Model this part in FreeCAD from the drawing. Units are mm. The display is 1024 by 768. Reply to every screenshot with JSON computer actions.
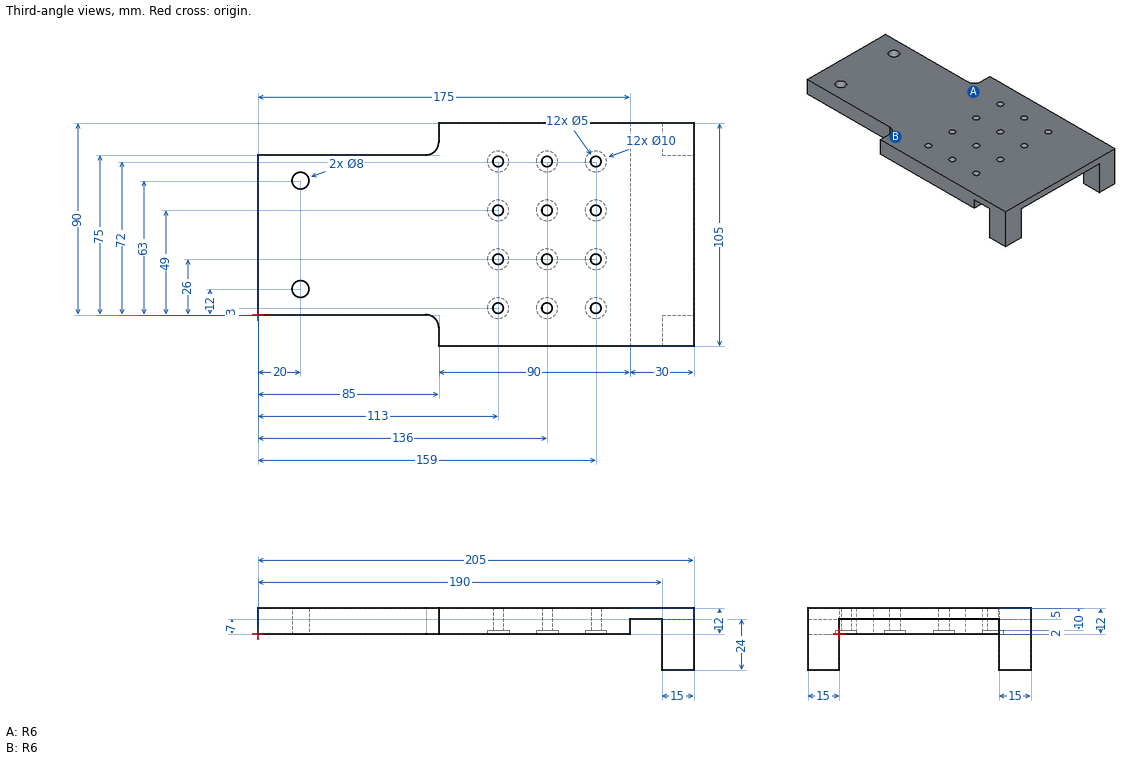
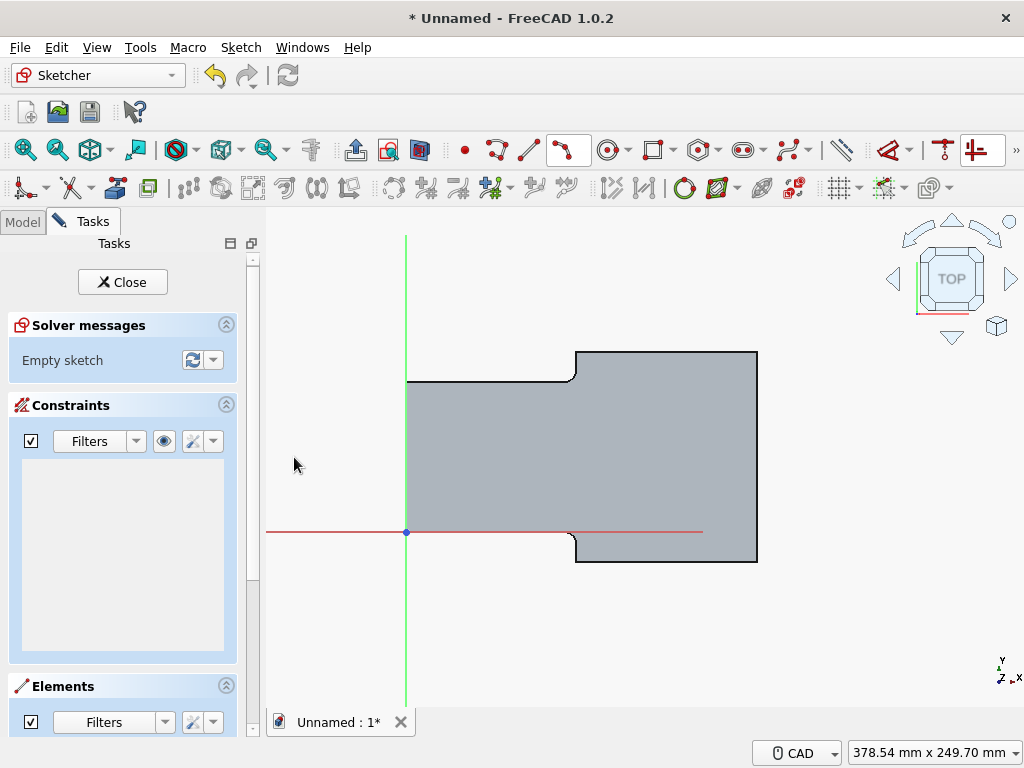
{"action": "left_click", "coordinate": [654, 150]}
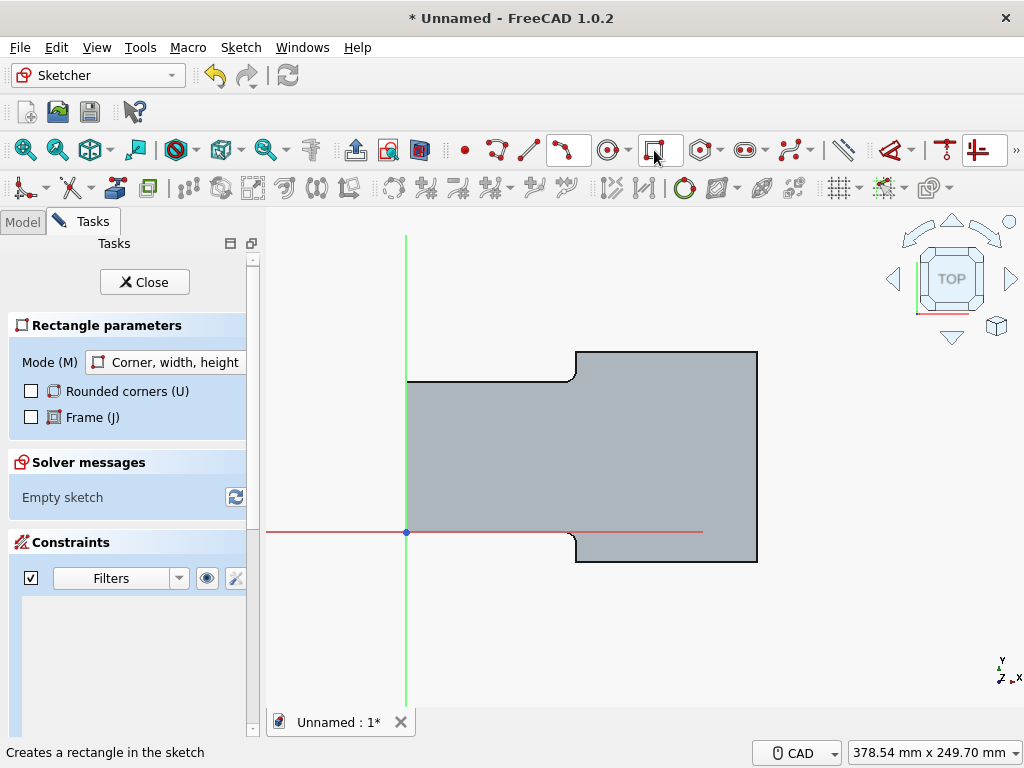
{"action": "left_click", "coordinate": [757, 352]}
{"action": "mouse_move", "coordinate": [817, 562]}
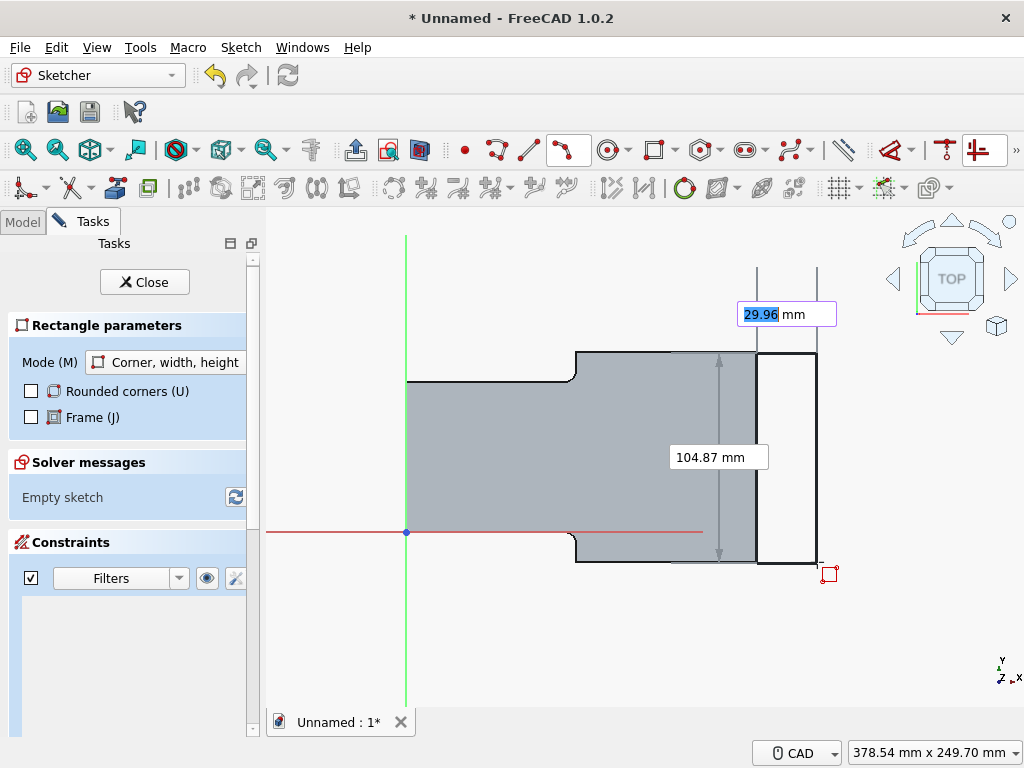
{"action": "type", "text": "30"}
{"action": "key", "text": "Tab"}
{"action": "type", "text": "105"}
{"action": "key", "text": "Return"}
{"action": "key", "text": "Escape"}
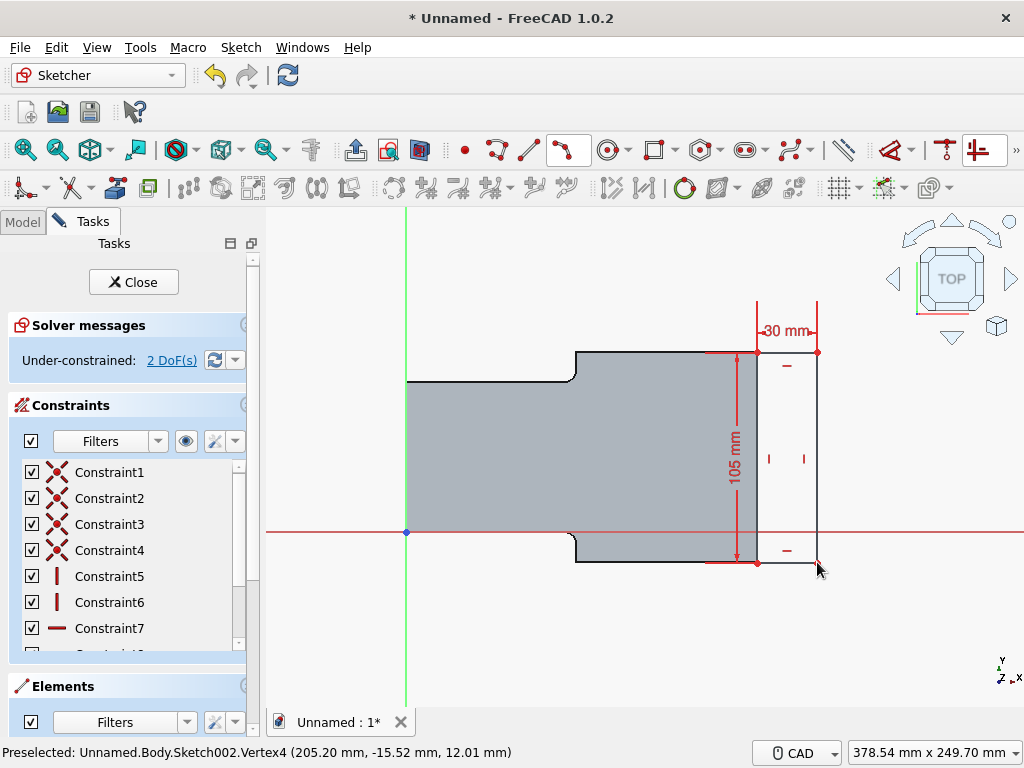
{"action": "left_click", "coordinate": [890, 150]}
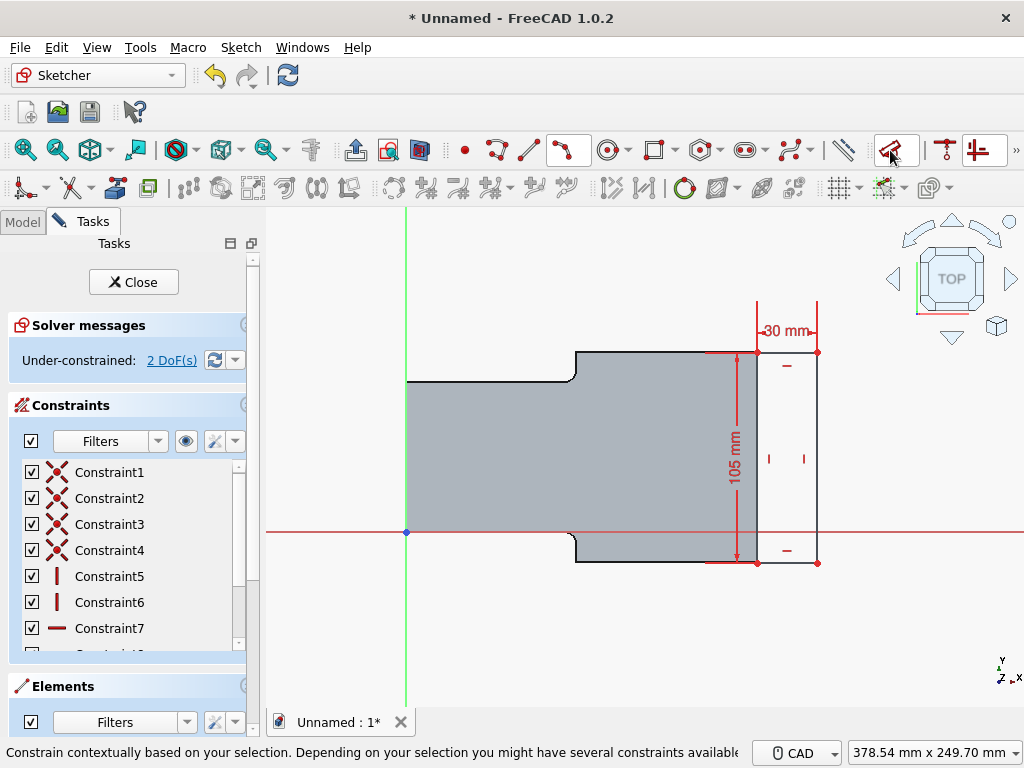
{"action": "left_click", "coordinate": [757, 353]}
{"action": "left_click", "coordinate": [372, 443]}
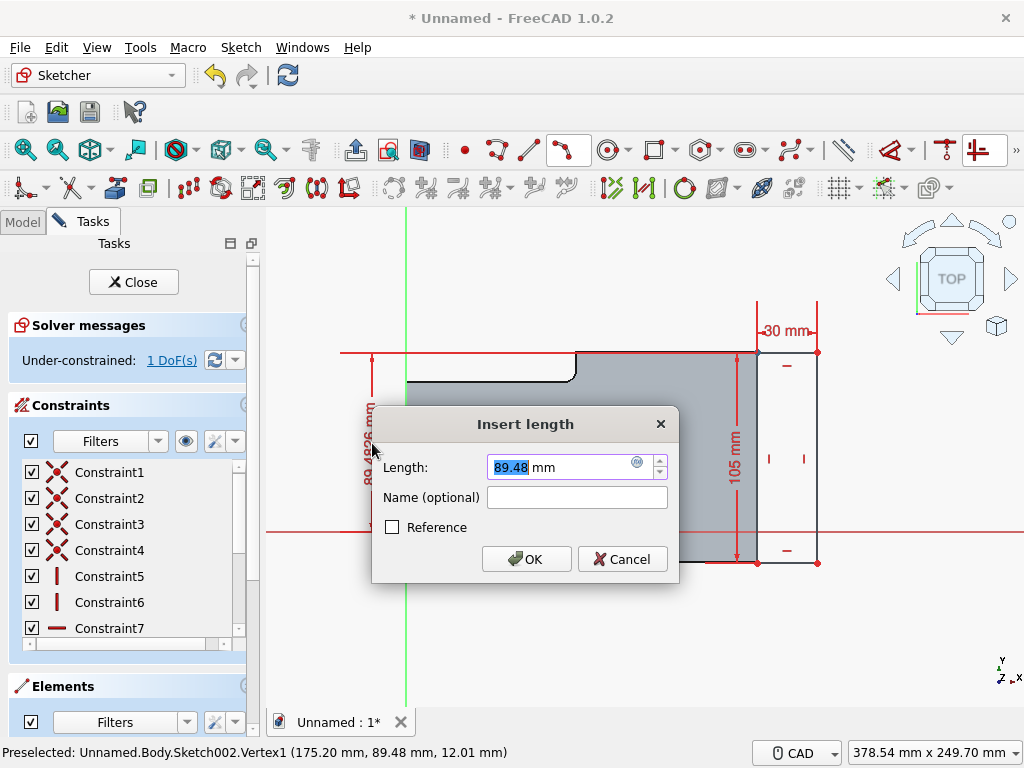
{"action": "type", "text": "90"}
{"action": "key", "text": "Return"}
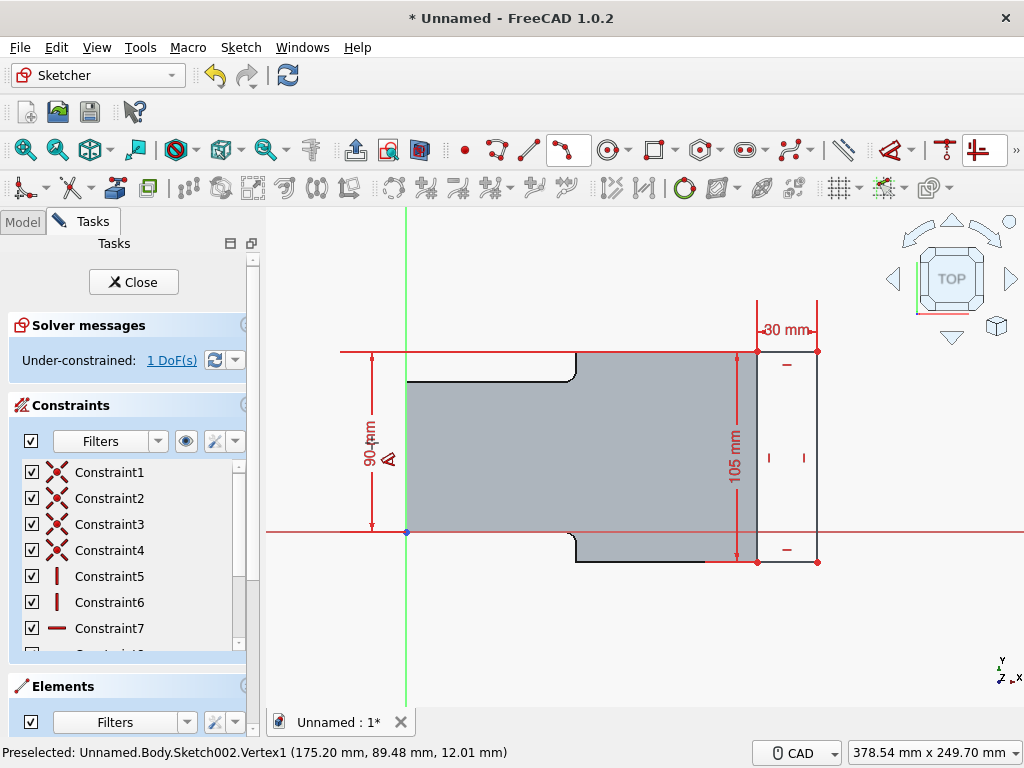
{"action": "left_click", "coordinate": [757, 352]}
{"action": "left_click", "coordinate": [582, 318]}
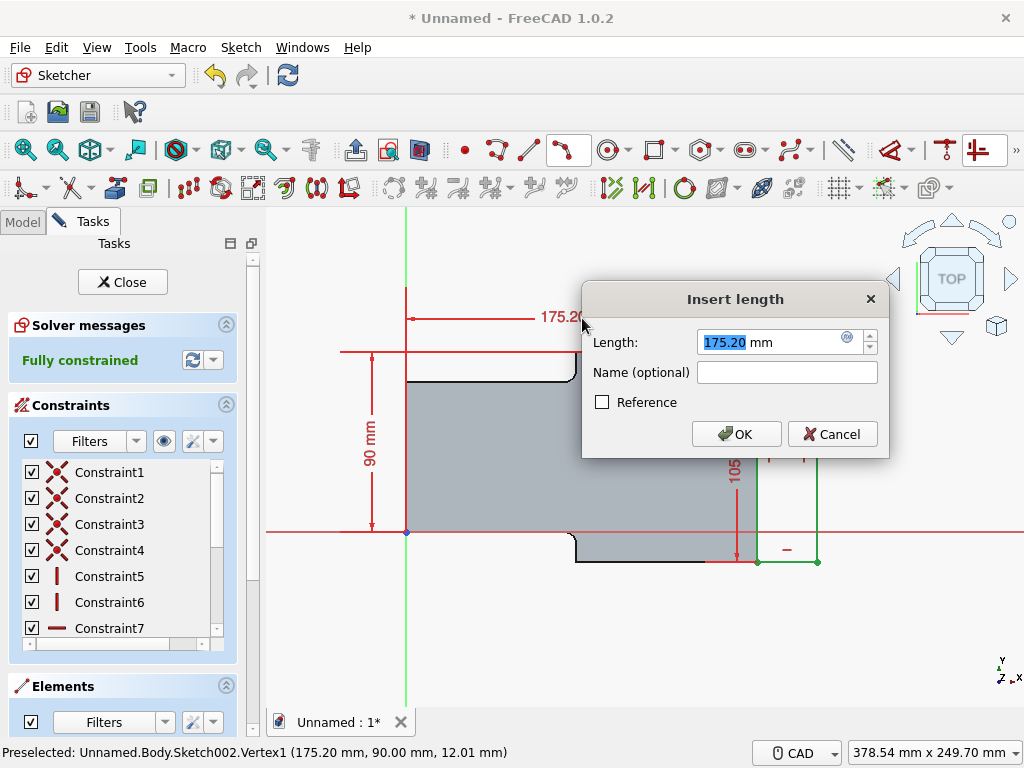
{"action": "type", "text": "175"}
{"action": "key", "text": "Return"}
{"action": "key", "text": "Escape"}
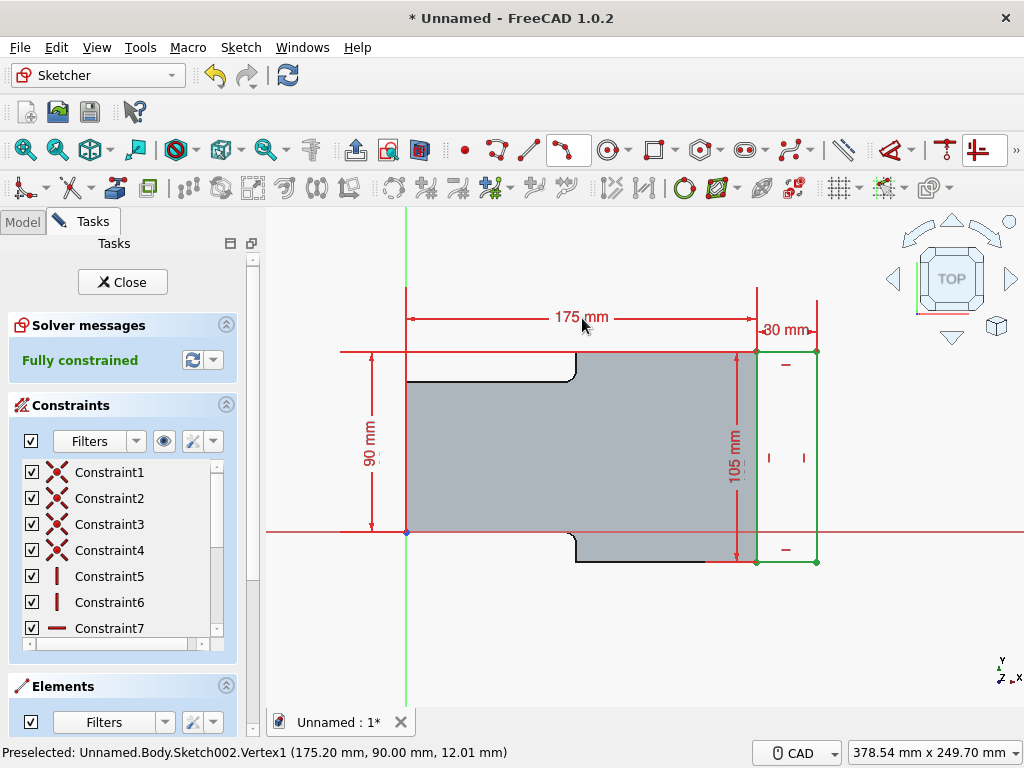
{"action": "left_click", "coordinate": [123, 282]}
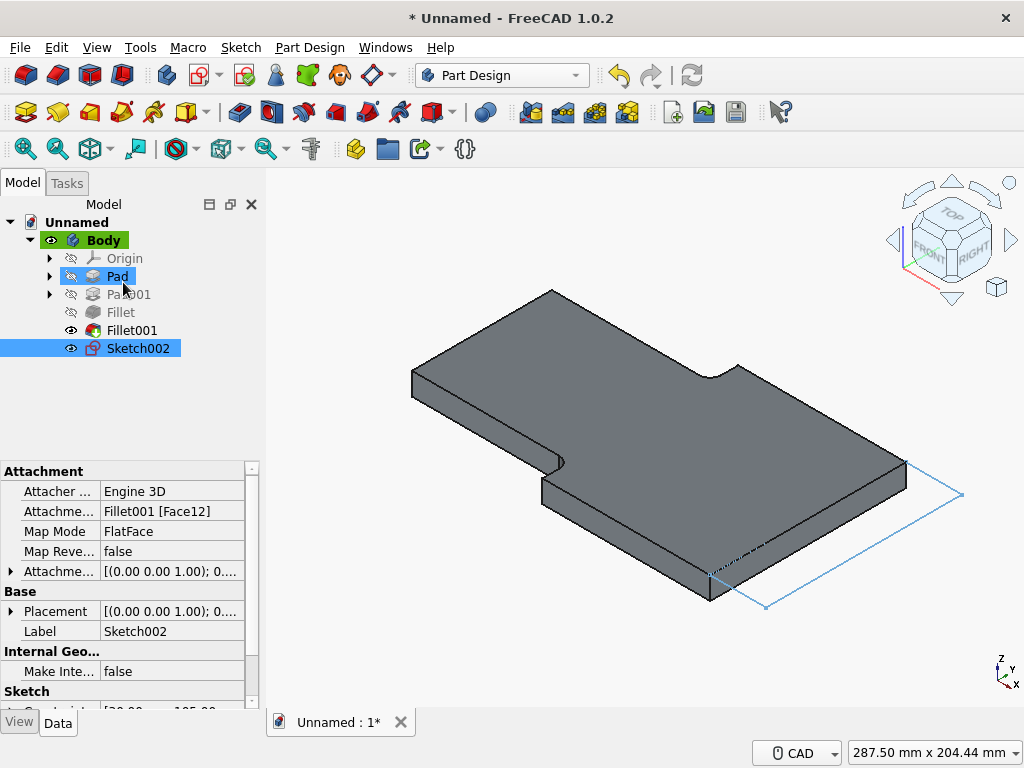
{"action": "left_click", "coordinate": [26, 112]}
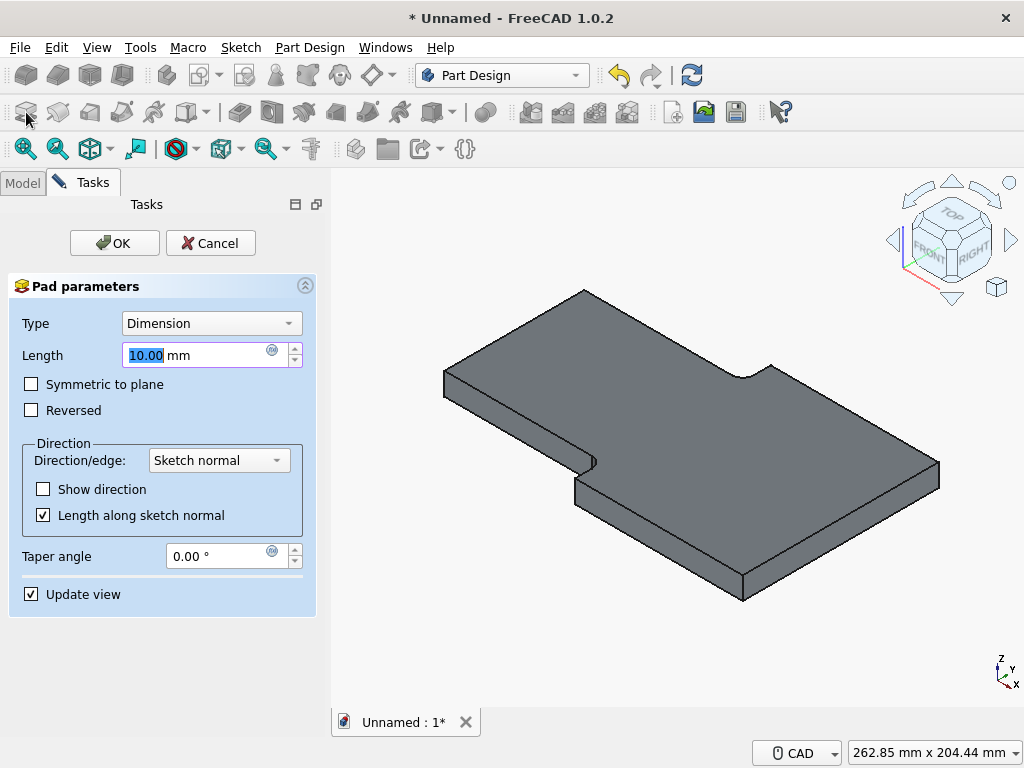
{"action": "type", "text": "5"}
{"action": "key", "text": "Tab"}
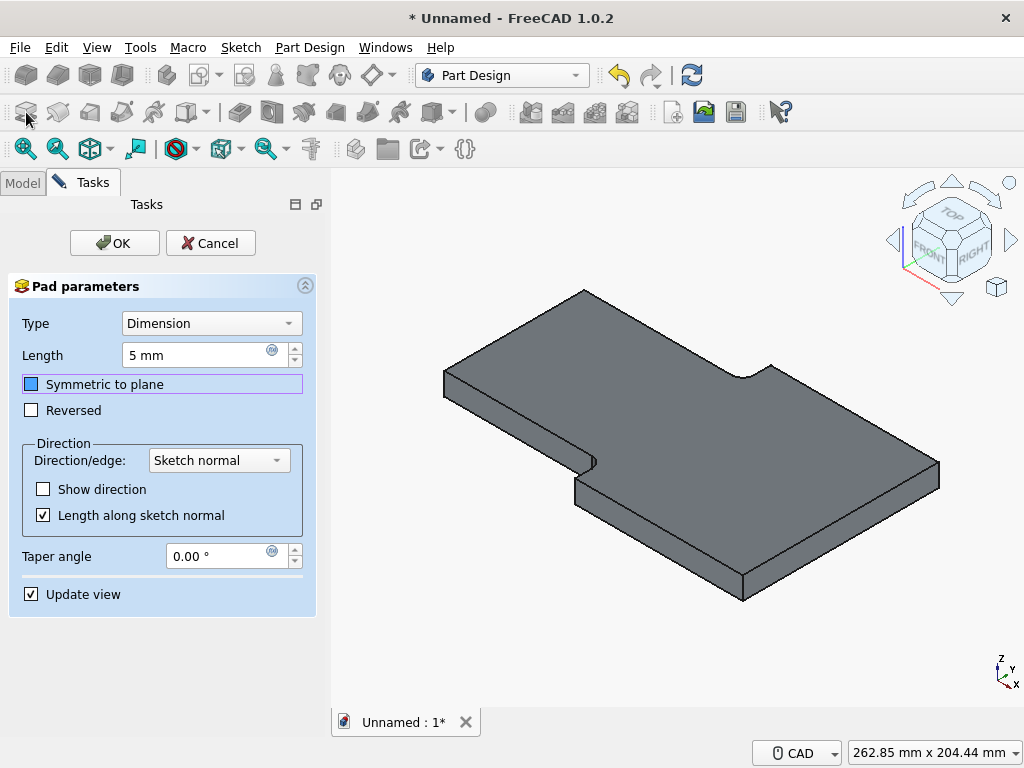
{"action": "left_click", "coordinate": [30, 410]}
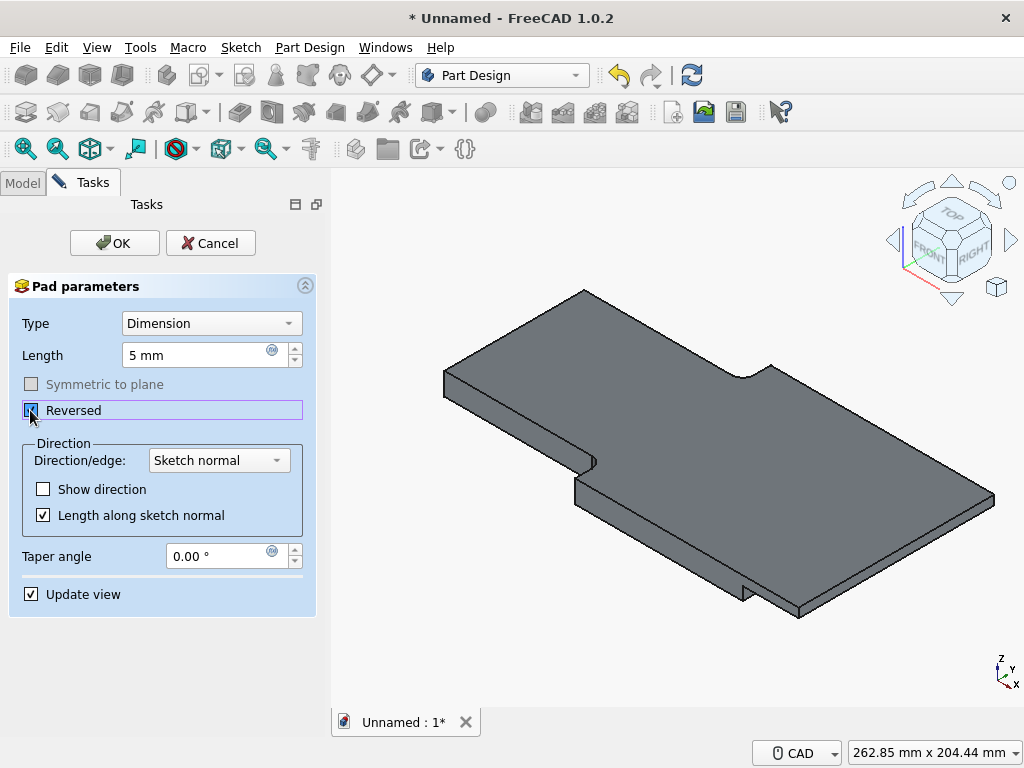
{"action": "left_click", "coordinate": [115, 243]}